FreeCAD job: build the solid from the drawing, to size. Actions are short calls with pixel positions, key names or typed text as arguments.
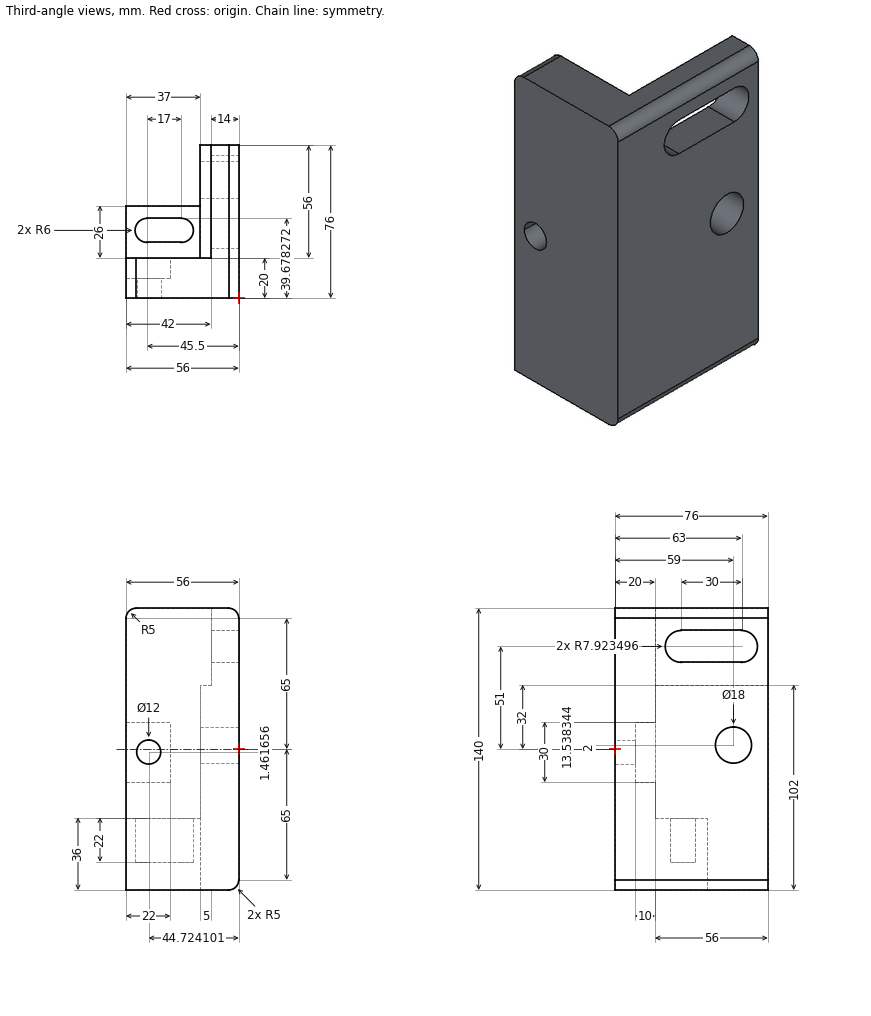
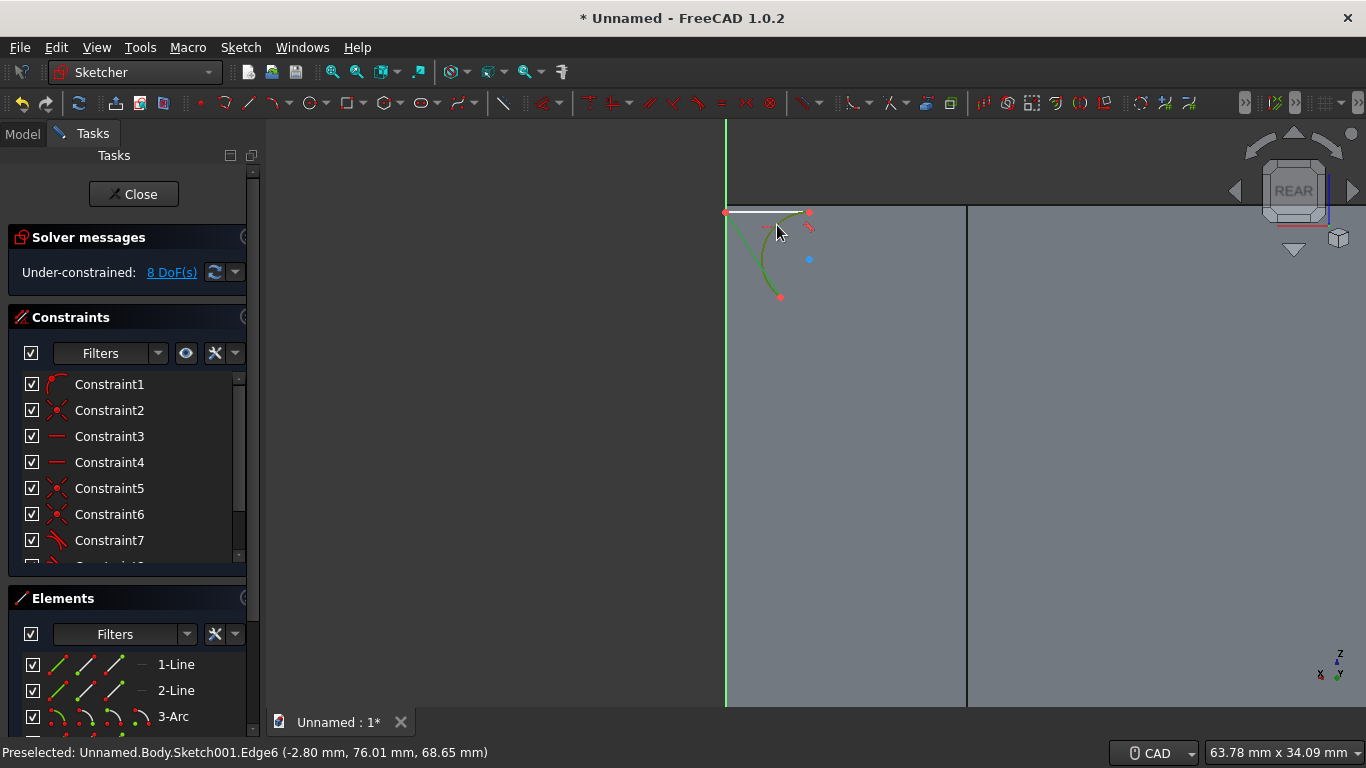
click(698, 104)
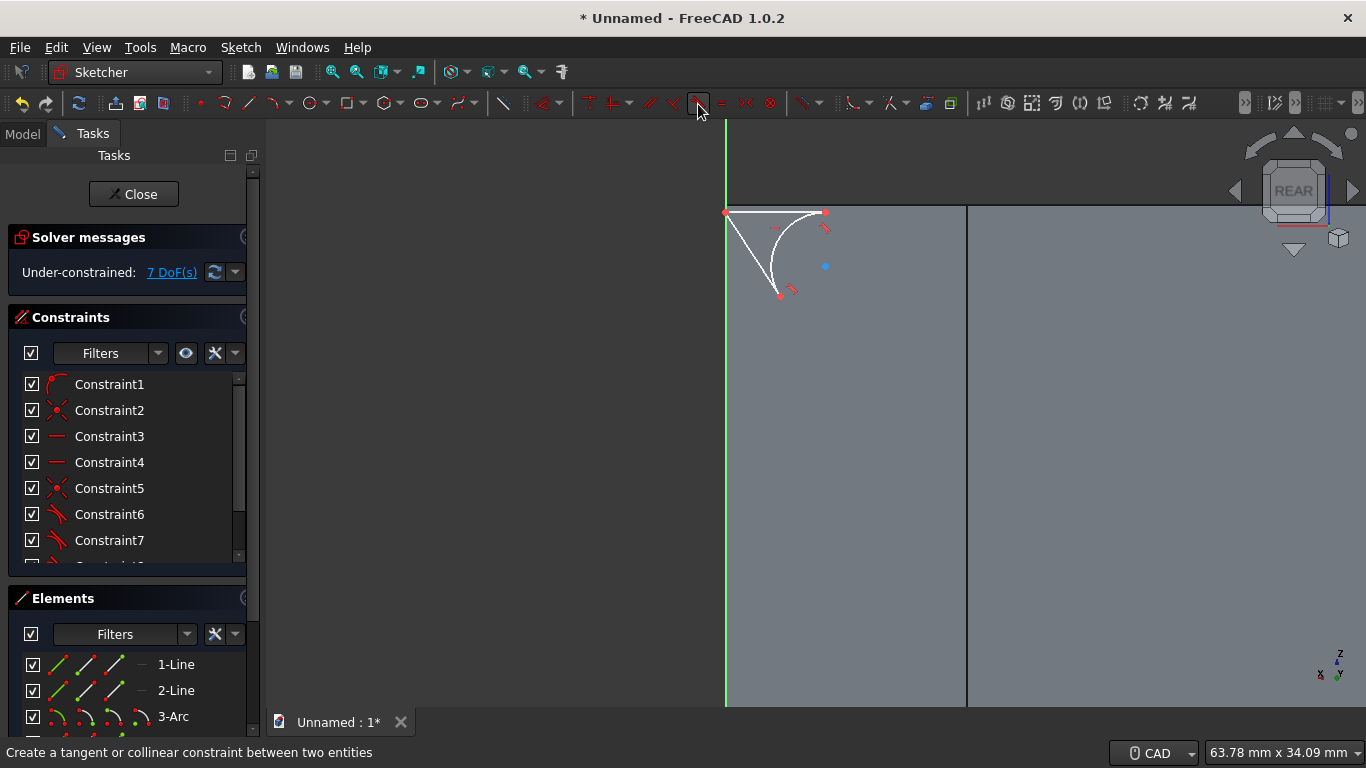
scroll(743, 215, down, 9)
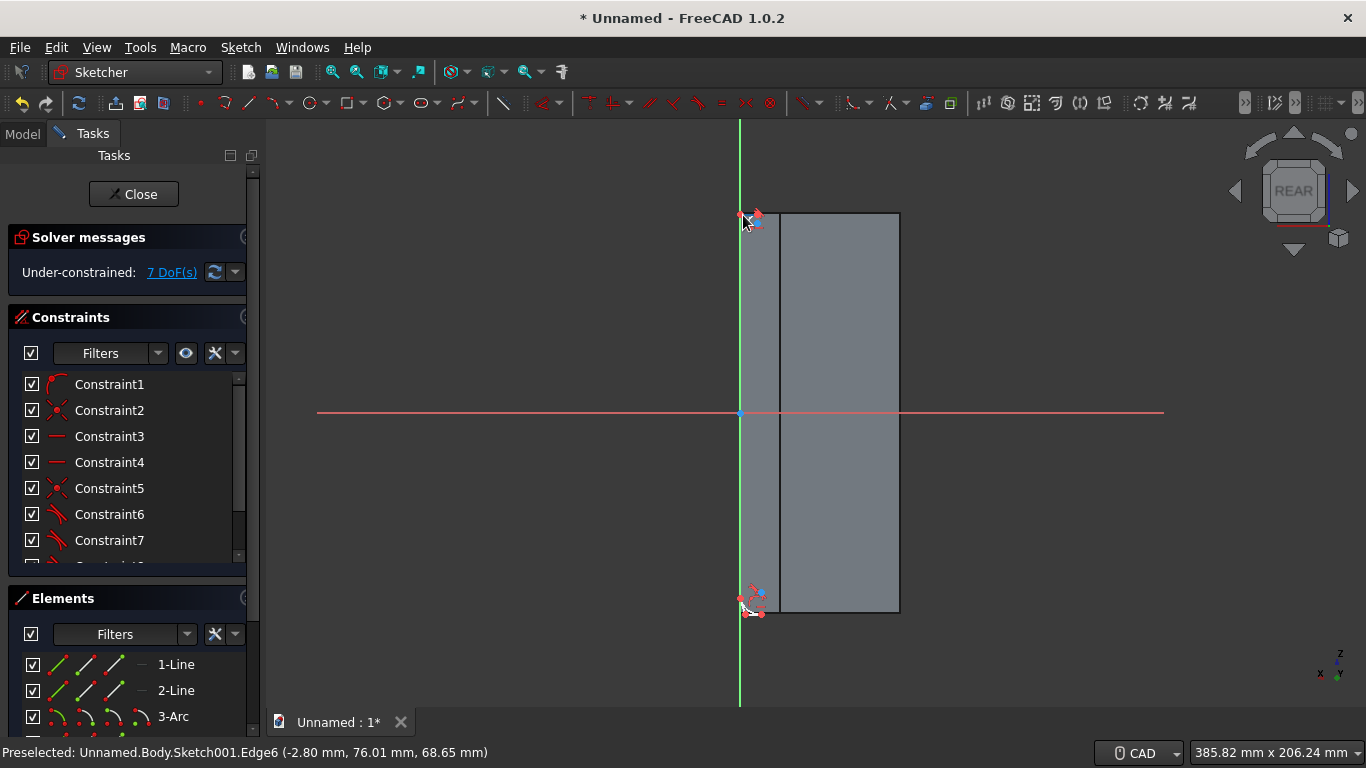
scroll(744, 610, up, 8)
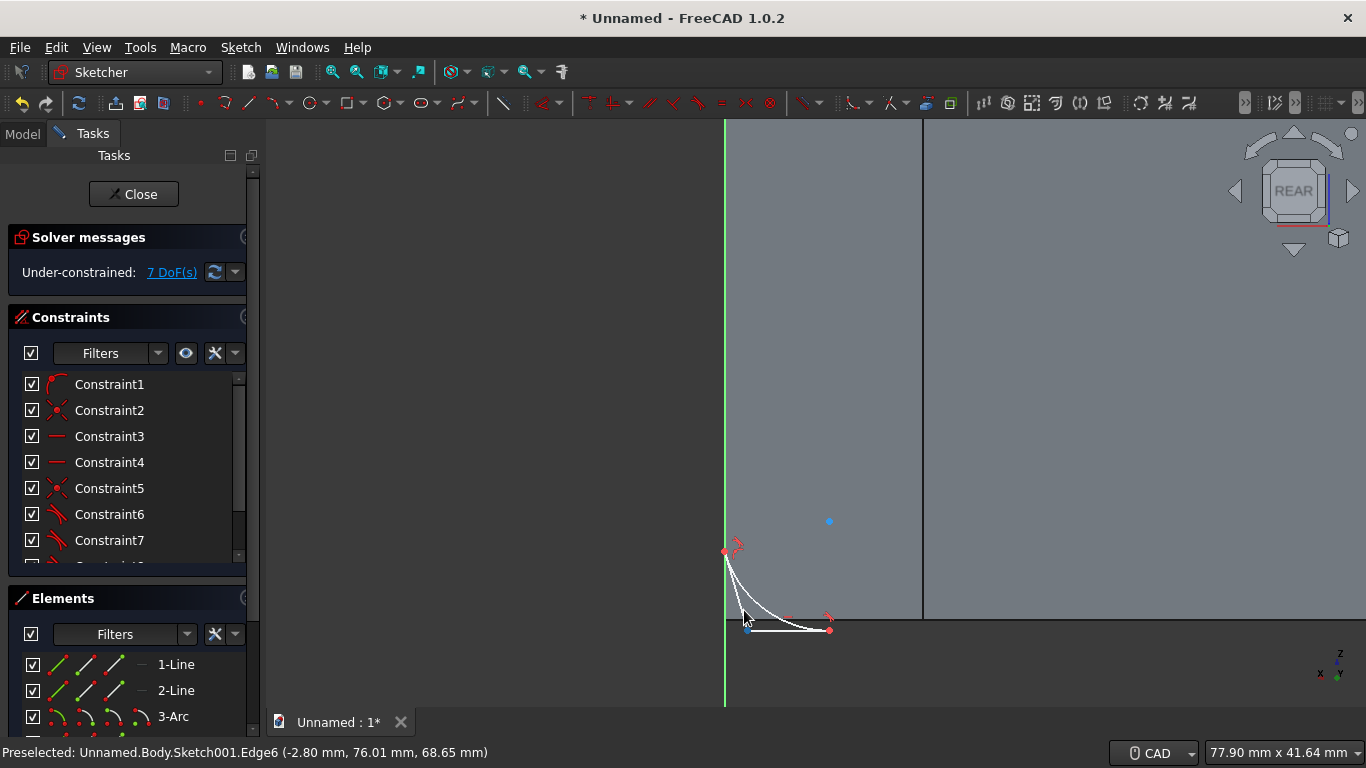
click(741, 607)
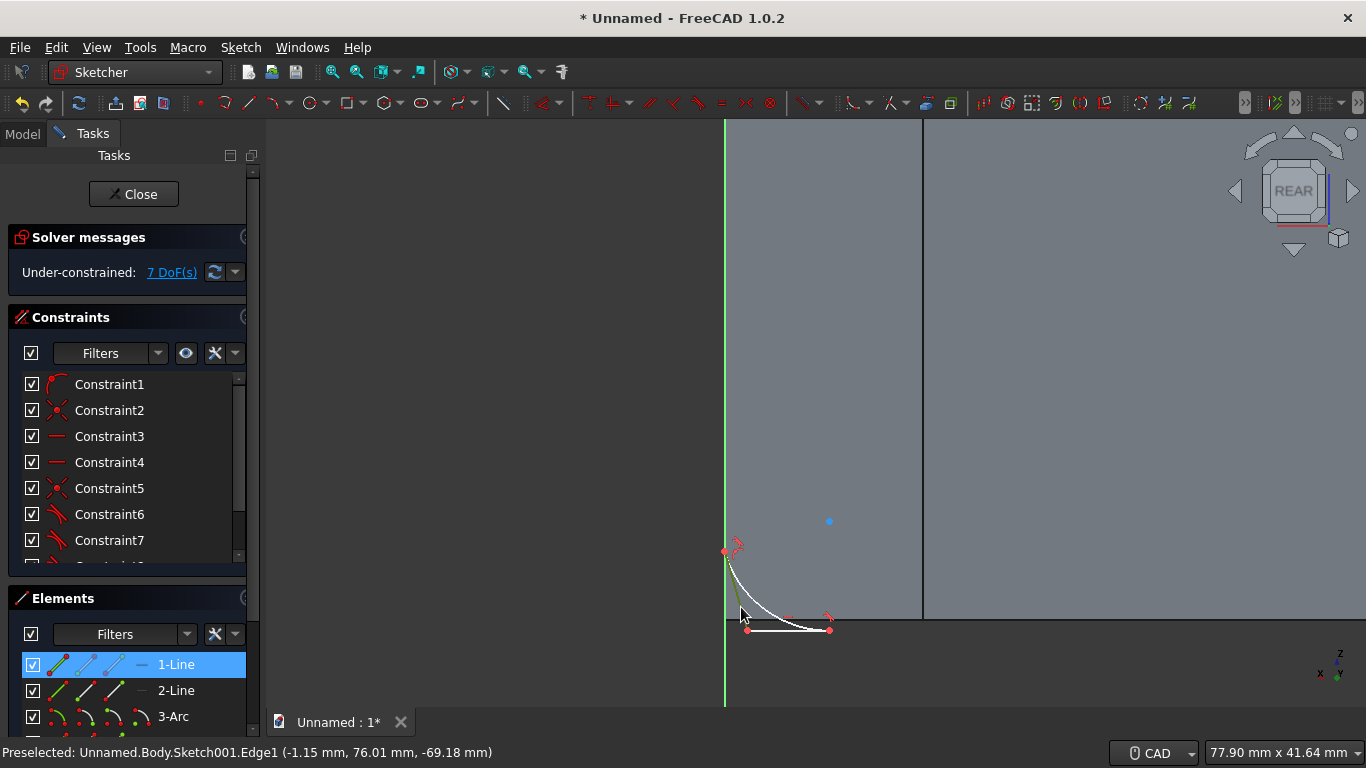
click(632, 104)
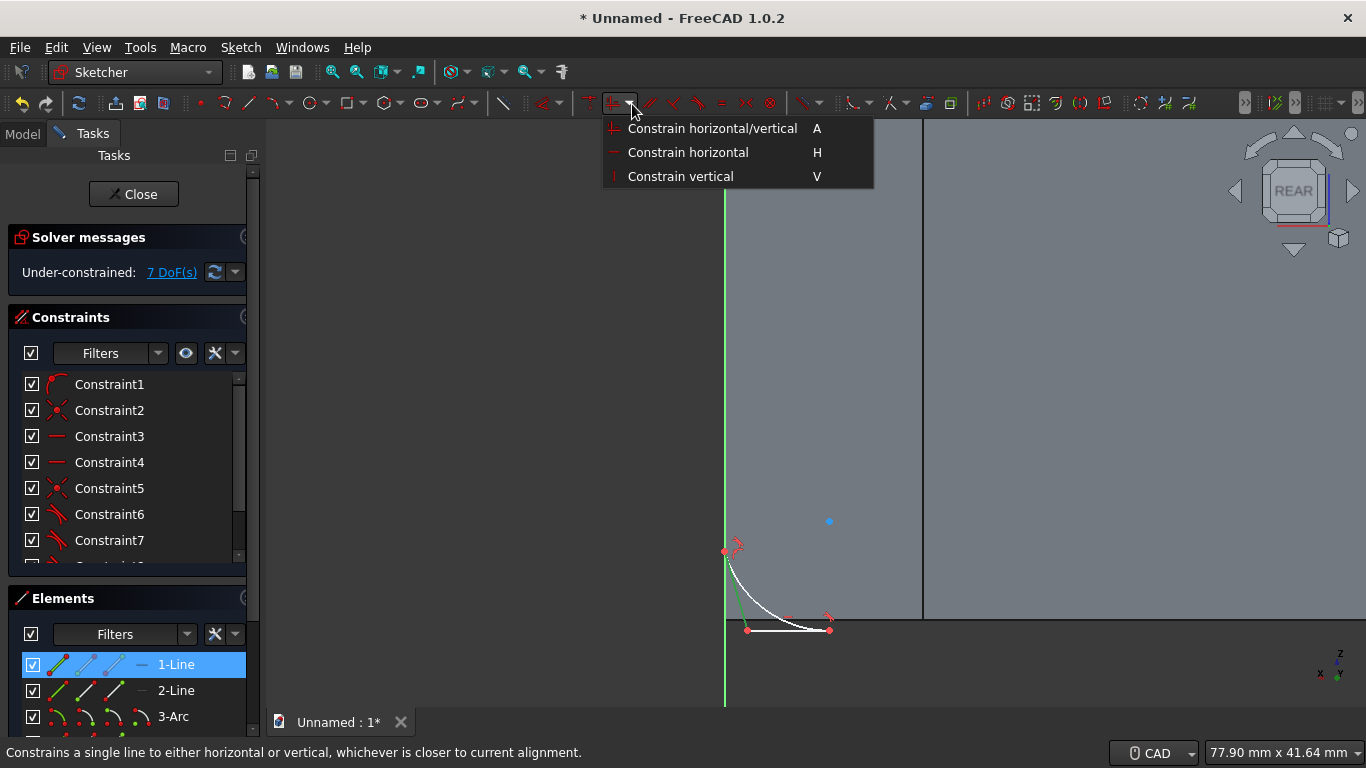
click(738, 176)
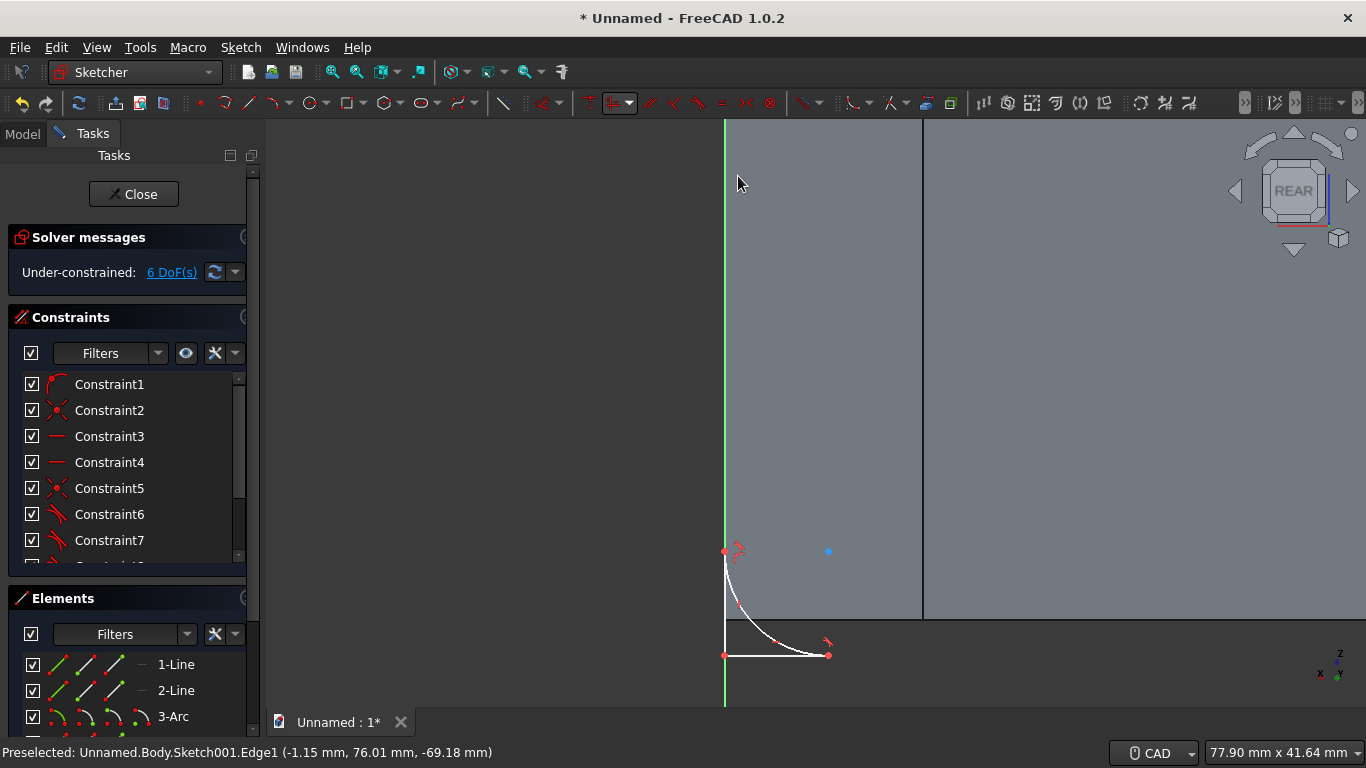
scroll(744, 611, down, 8)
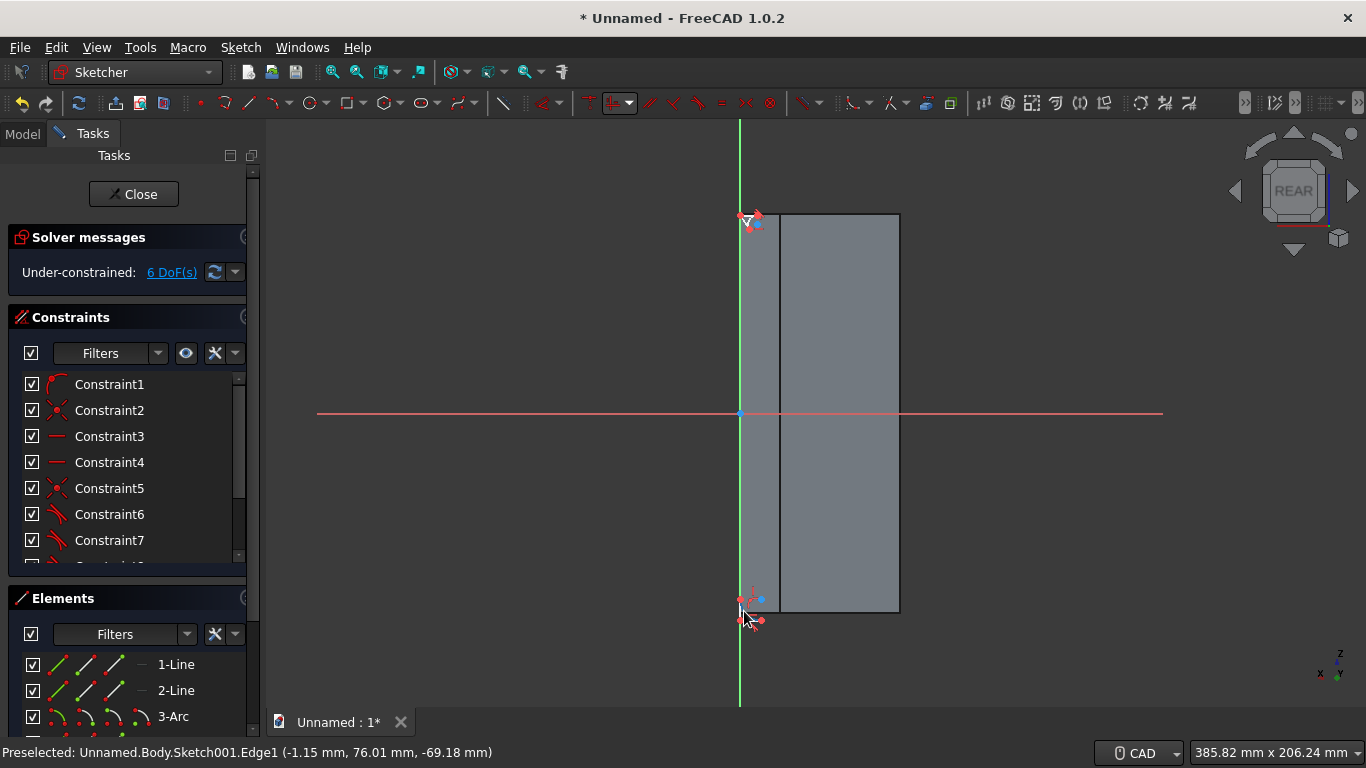
scroll(743, 220, up, 9)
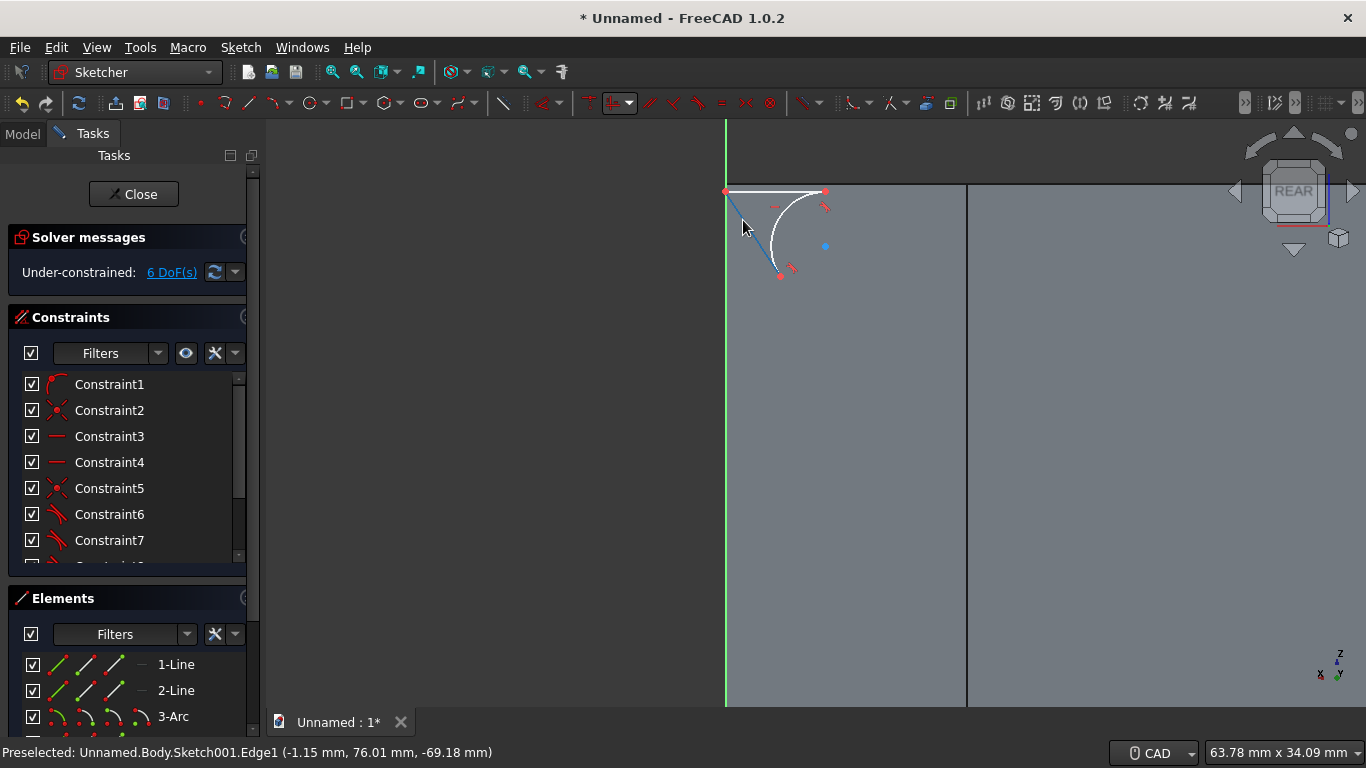
click(742, 217)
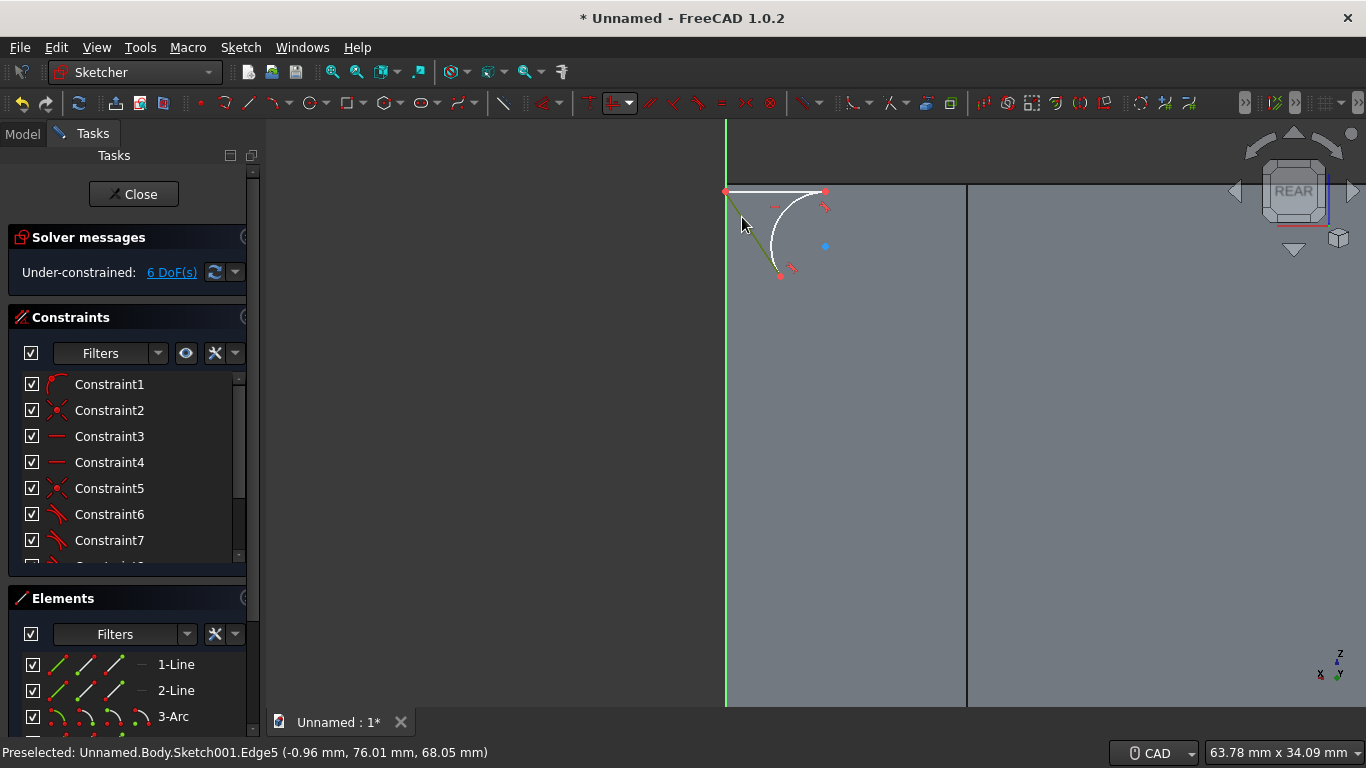
click(632, 104)